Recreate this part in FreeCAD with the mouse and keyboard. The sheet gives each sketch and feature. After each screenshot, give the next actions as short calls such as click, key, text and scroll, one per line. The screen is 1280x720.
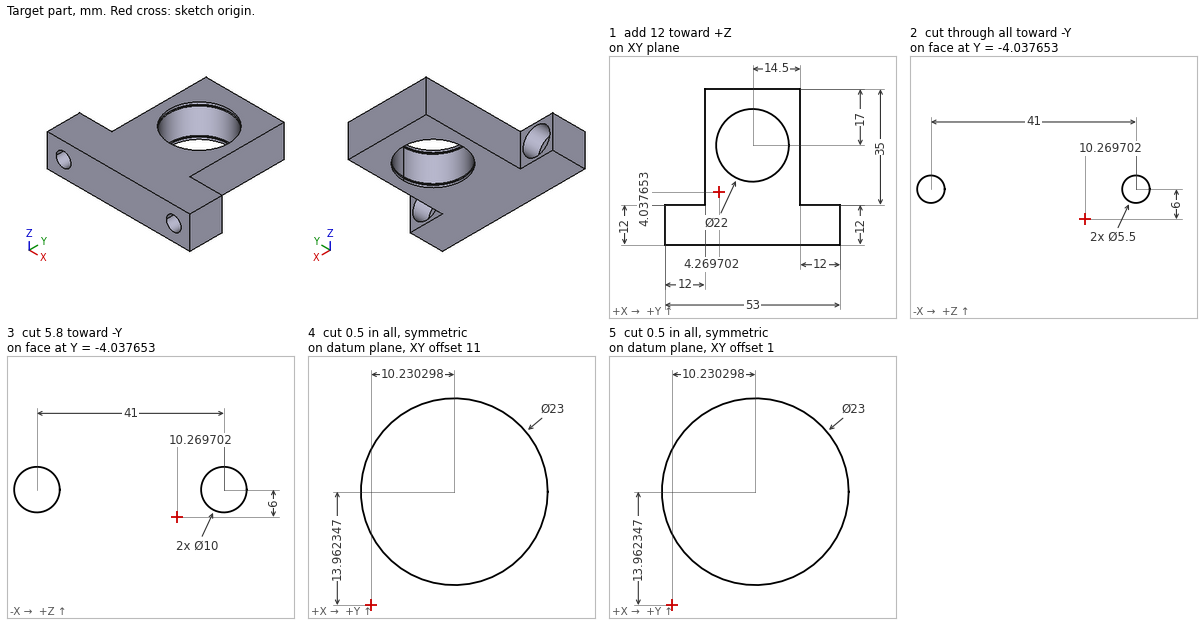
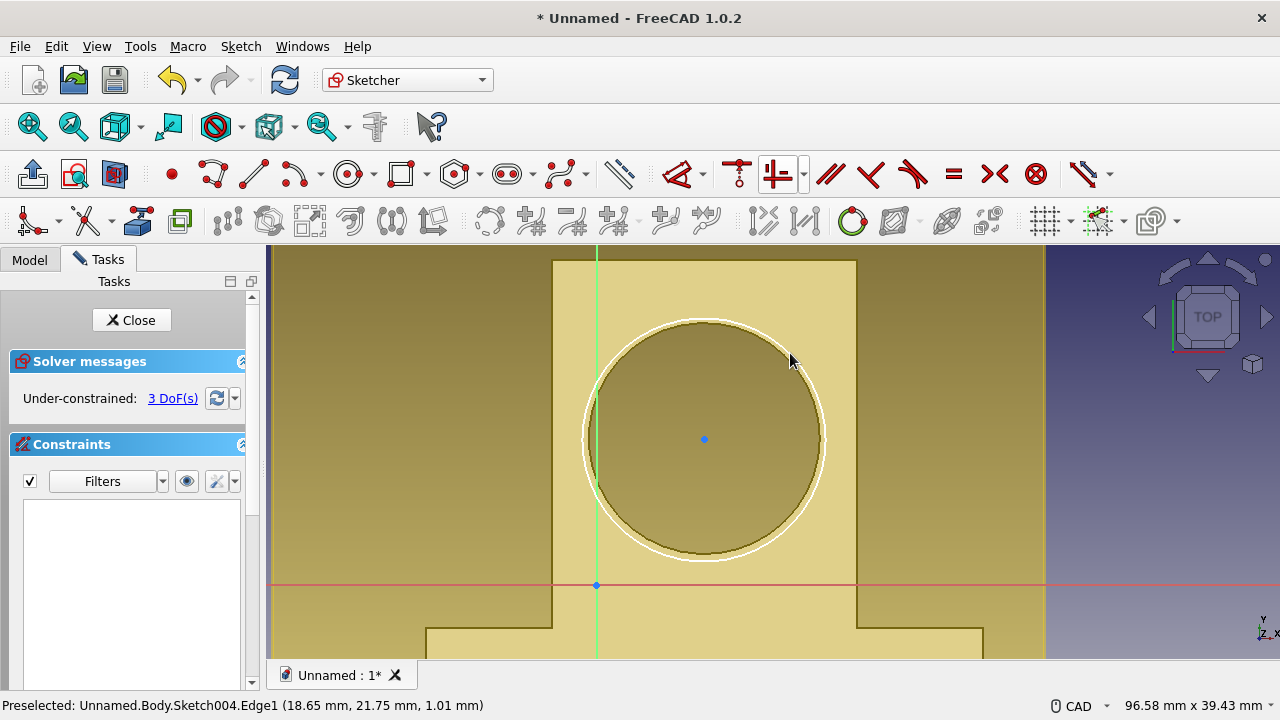
key(d)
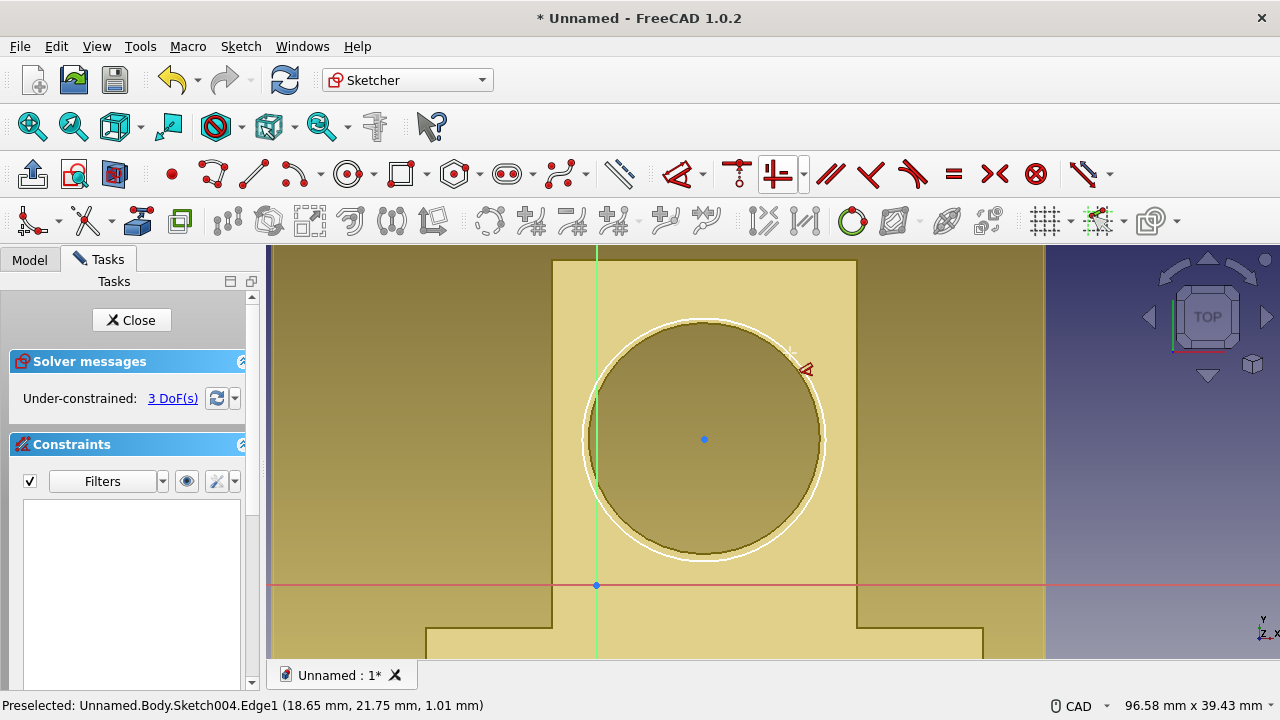
click(790, 354)
click(813, 331)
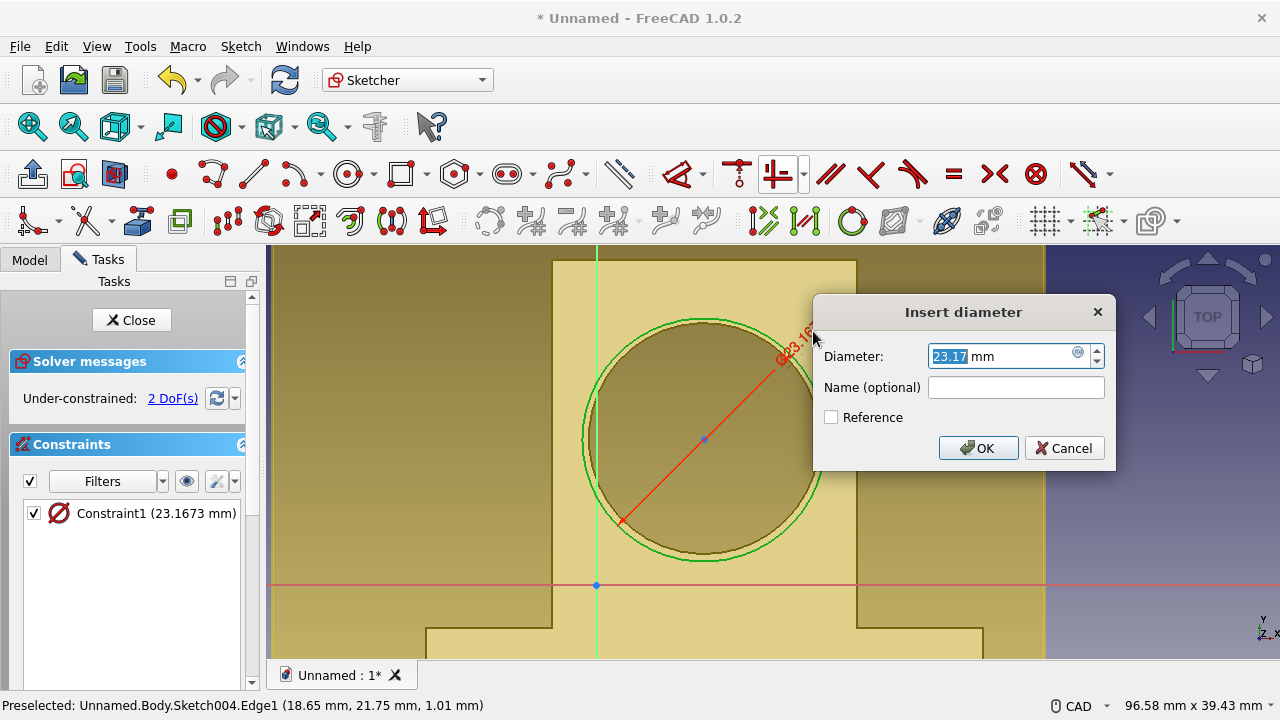
text(23)
key(Return)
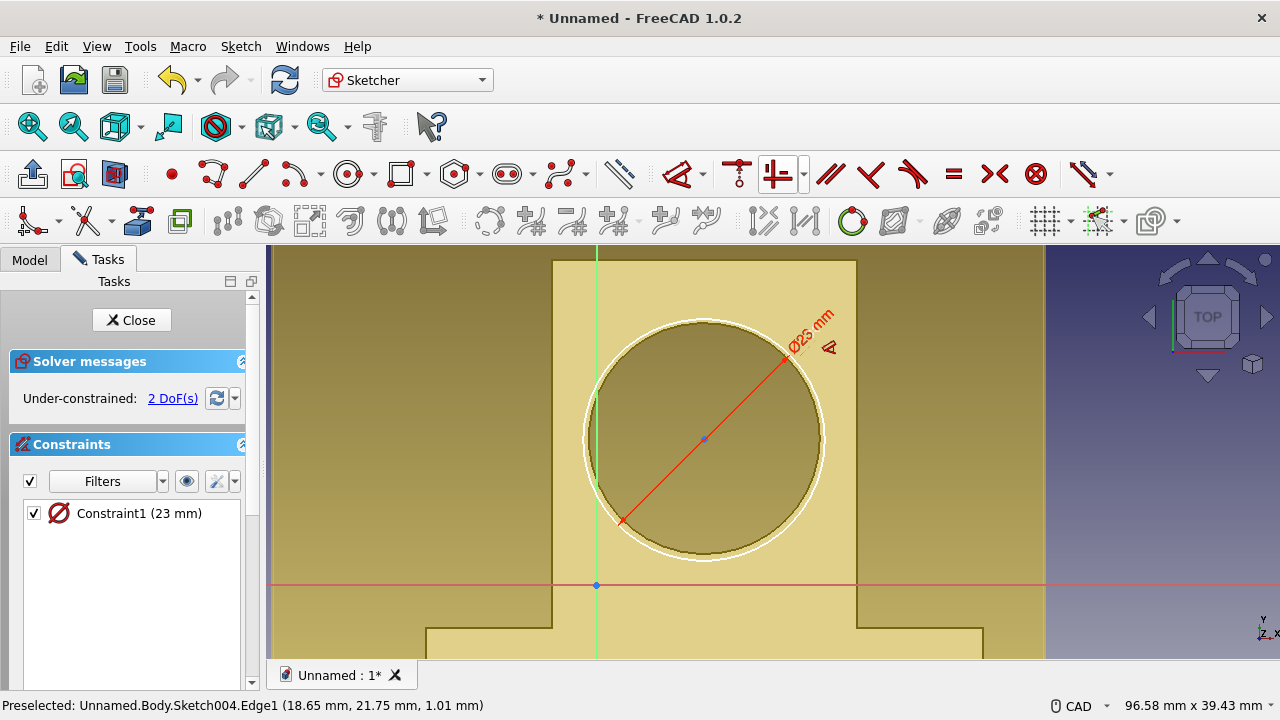
click(704, 440)
click(650, 619)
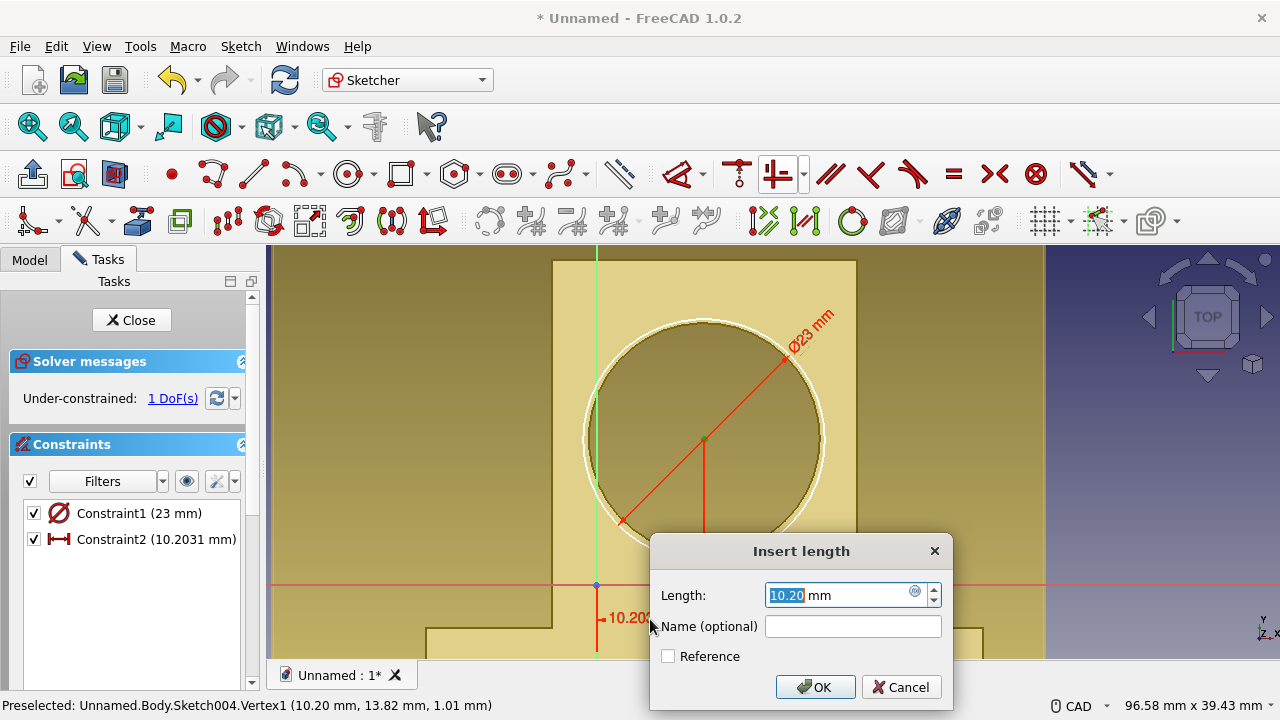
text(10.230298)
key(Return)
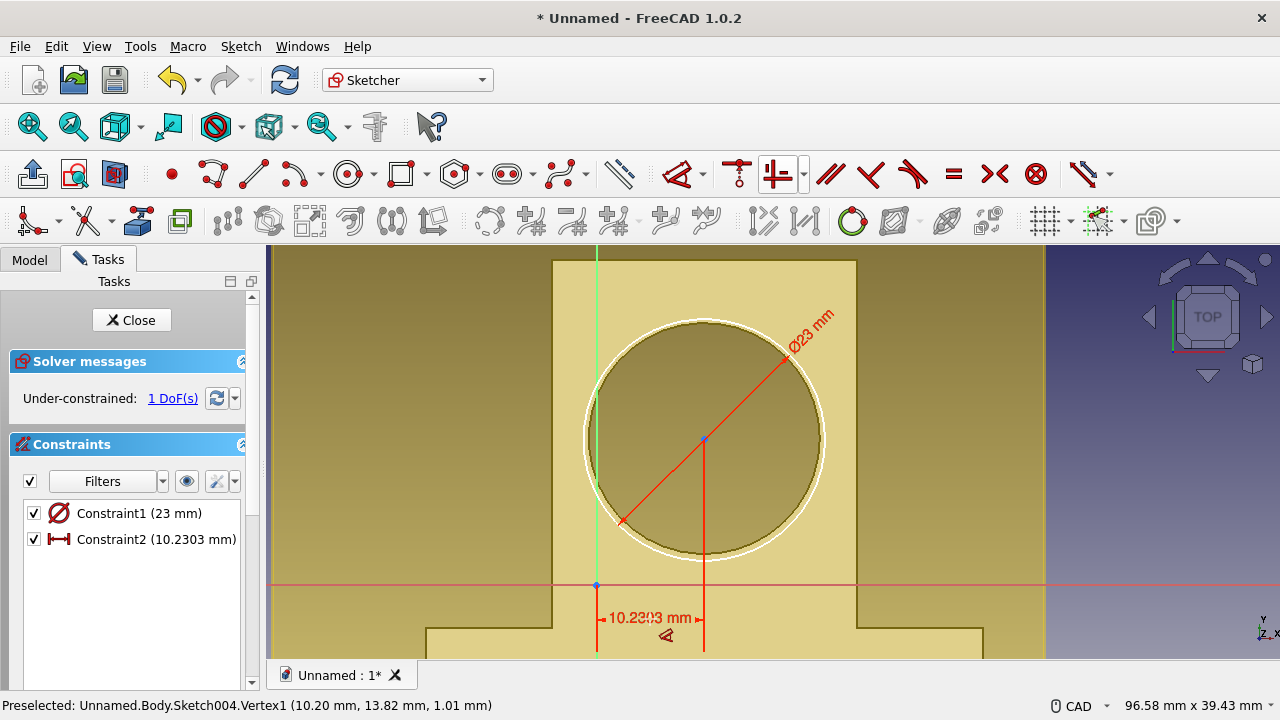
click(704, 440)
click(563, 513)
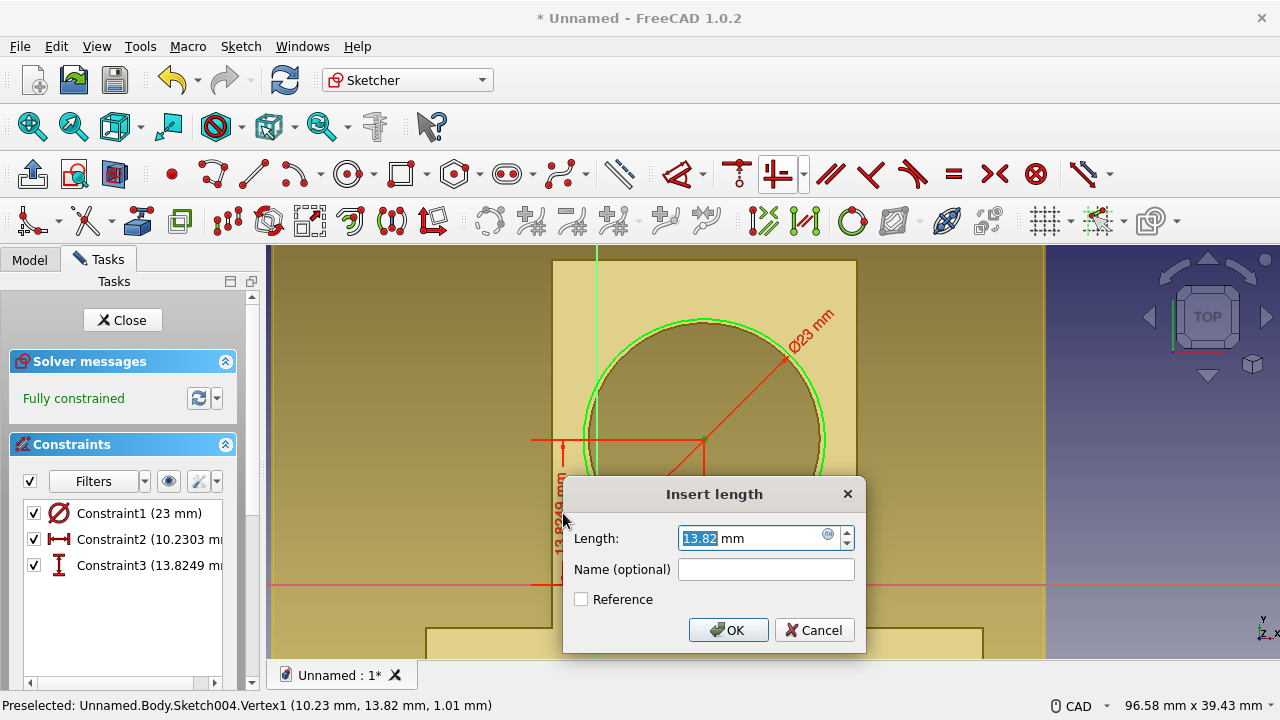
text(13.962347)
key(Return)
key(Escape)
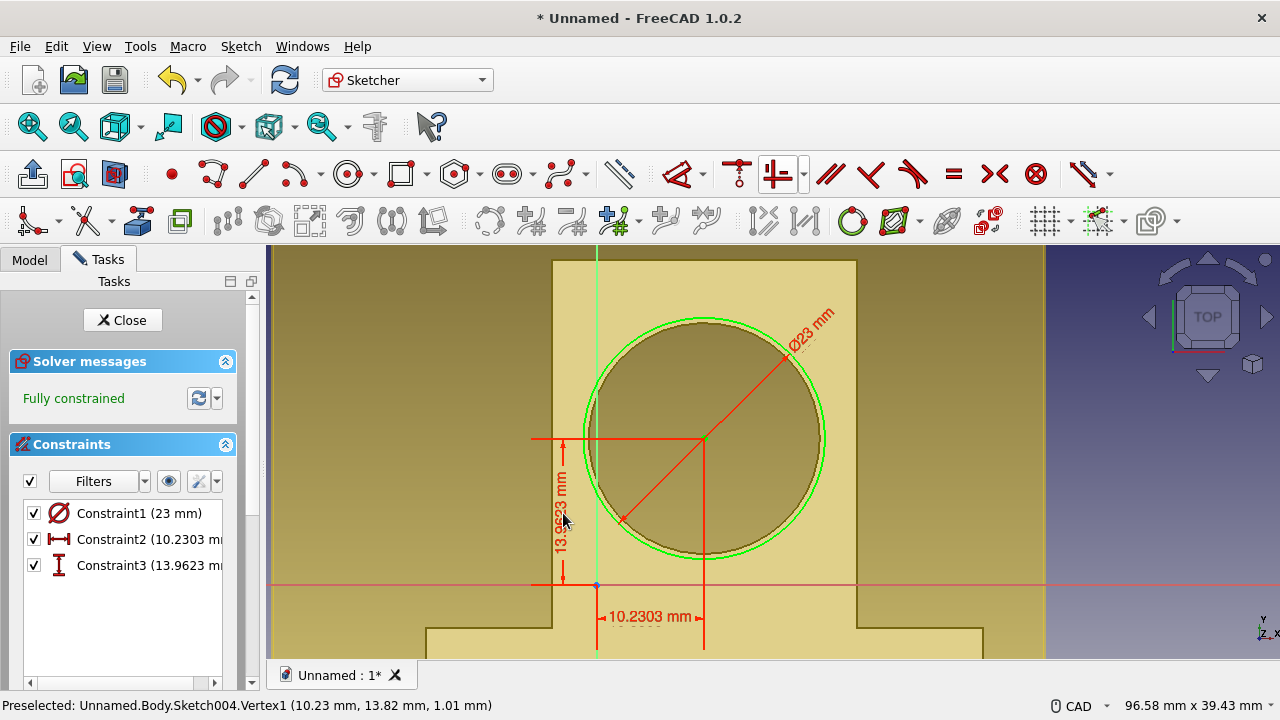
click(123, 320)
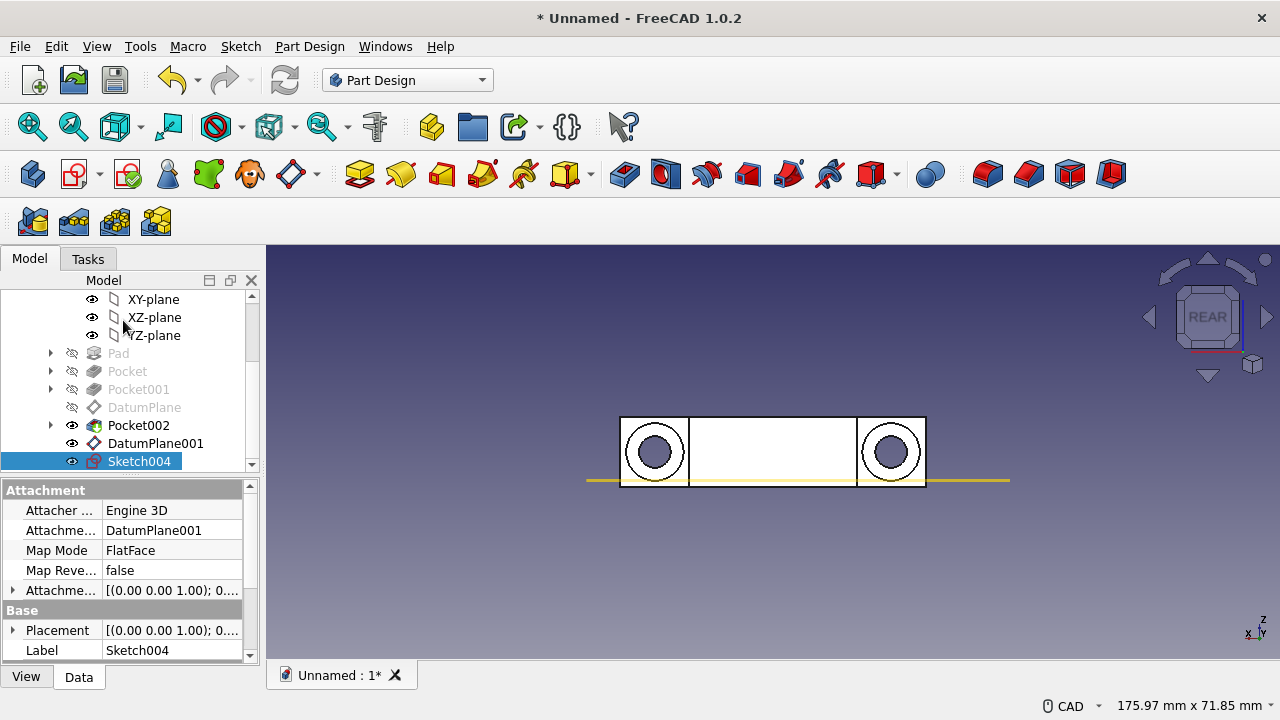
click(625, 174)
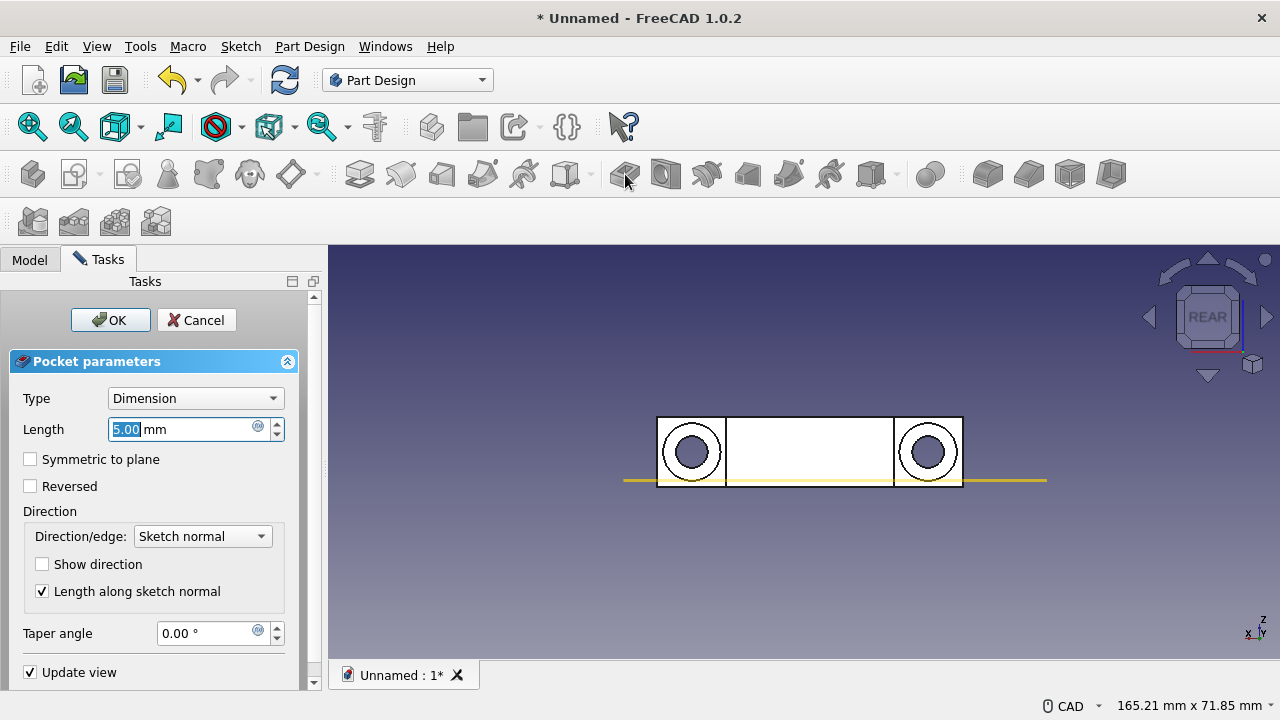
text(0.5)
key(Tab)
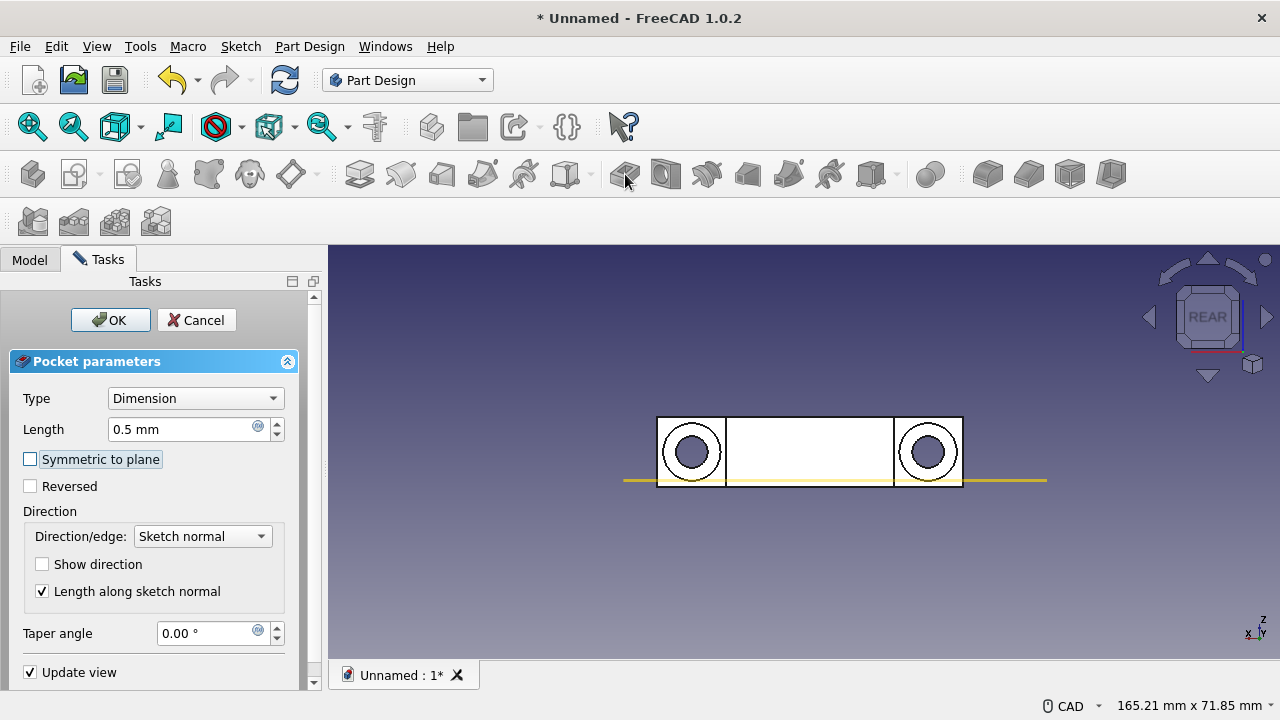
click(31, 459)